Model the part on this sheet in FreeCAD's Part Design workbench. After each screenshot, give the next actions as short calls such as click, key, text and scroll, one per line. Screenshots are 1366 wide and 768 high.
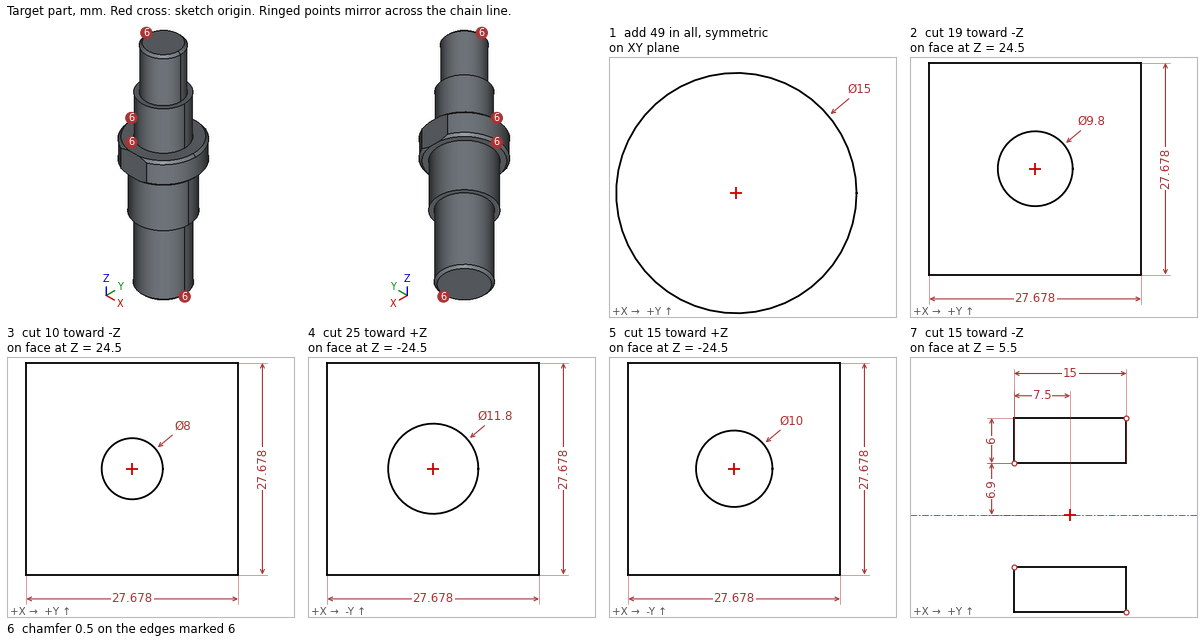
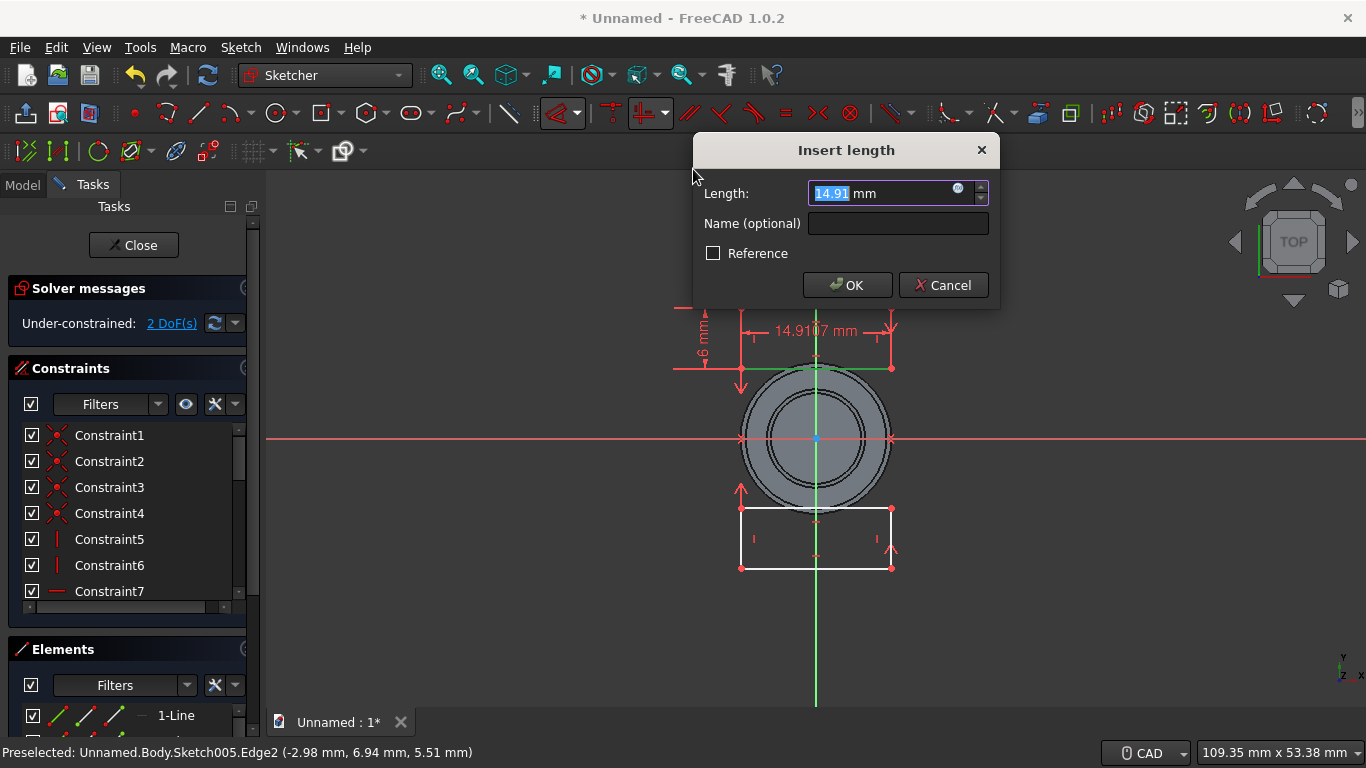
text(15)
key(Return)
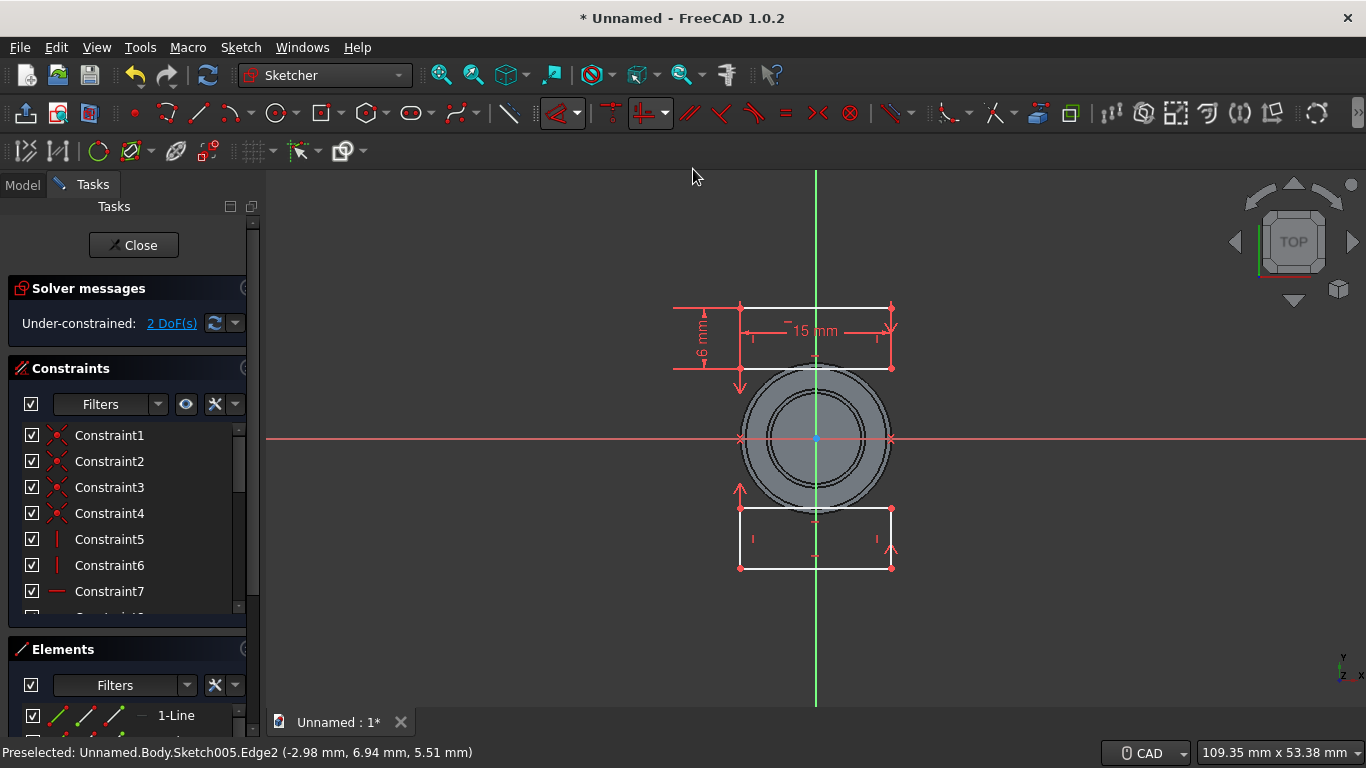
click(740, 308)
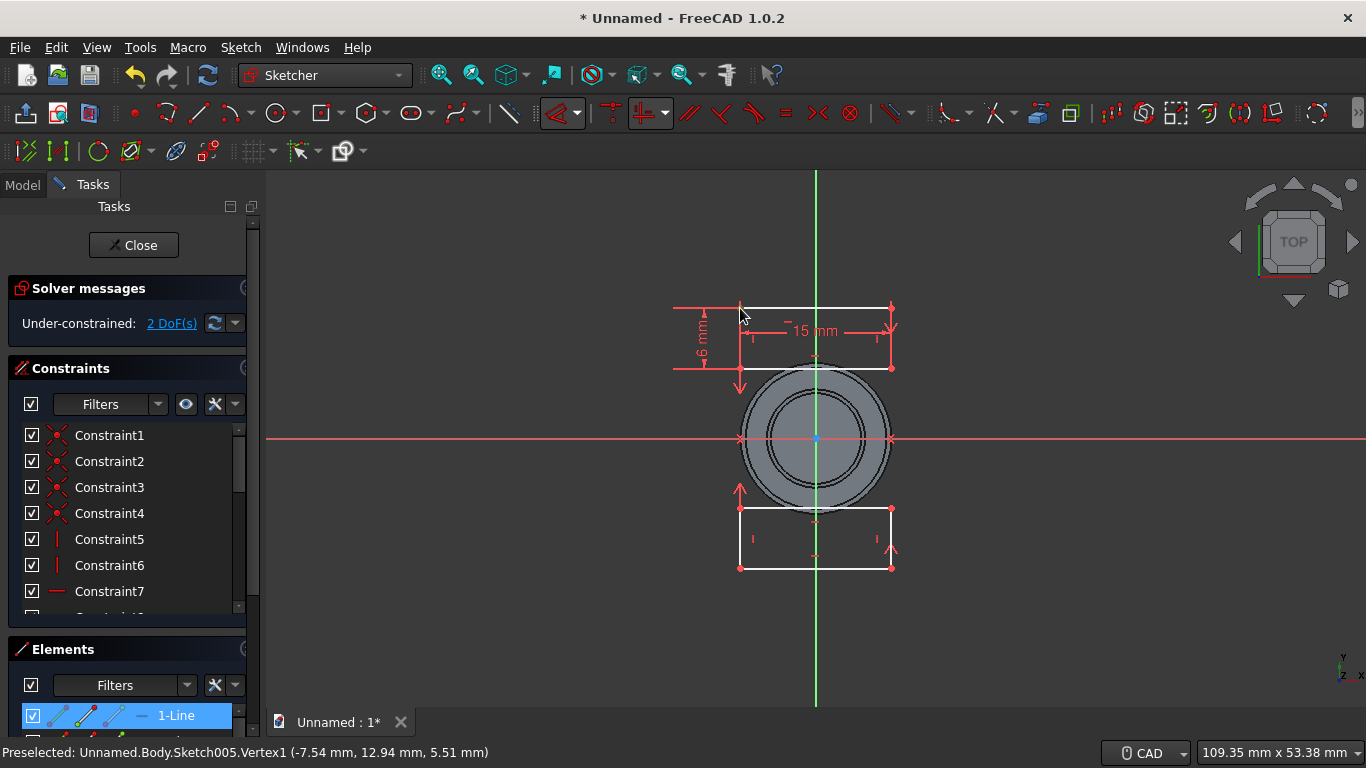
key(l)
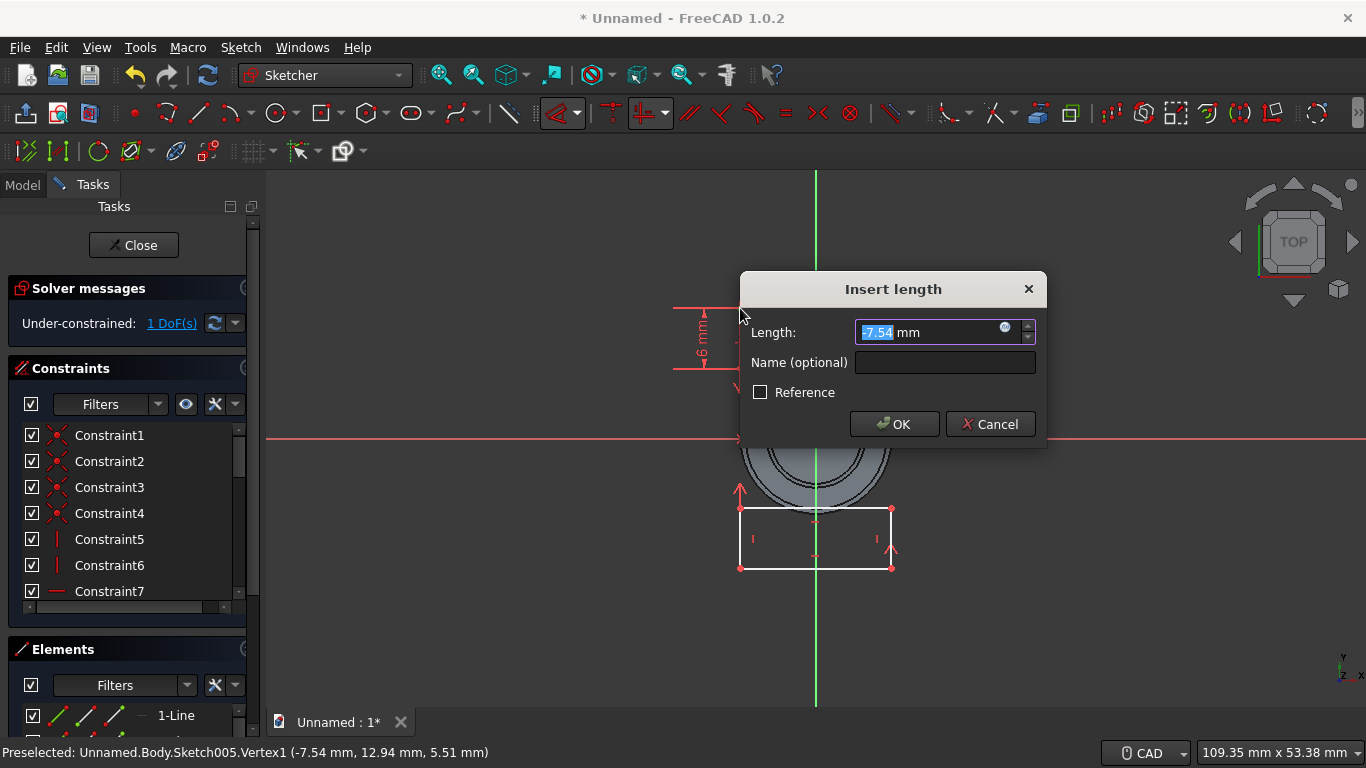
text(-7.5)
key(Return)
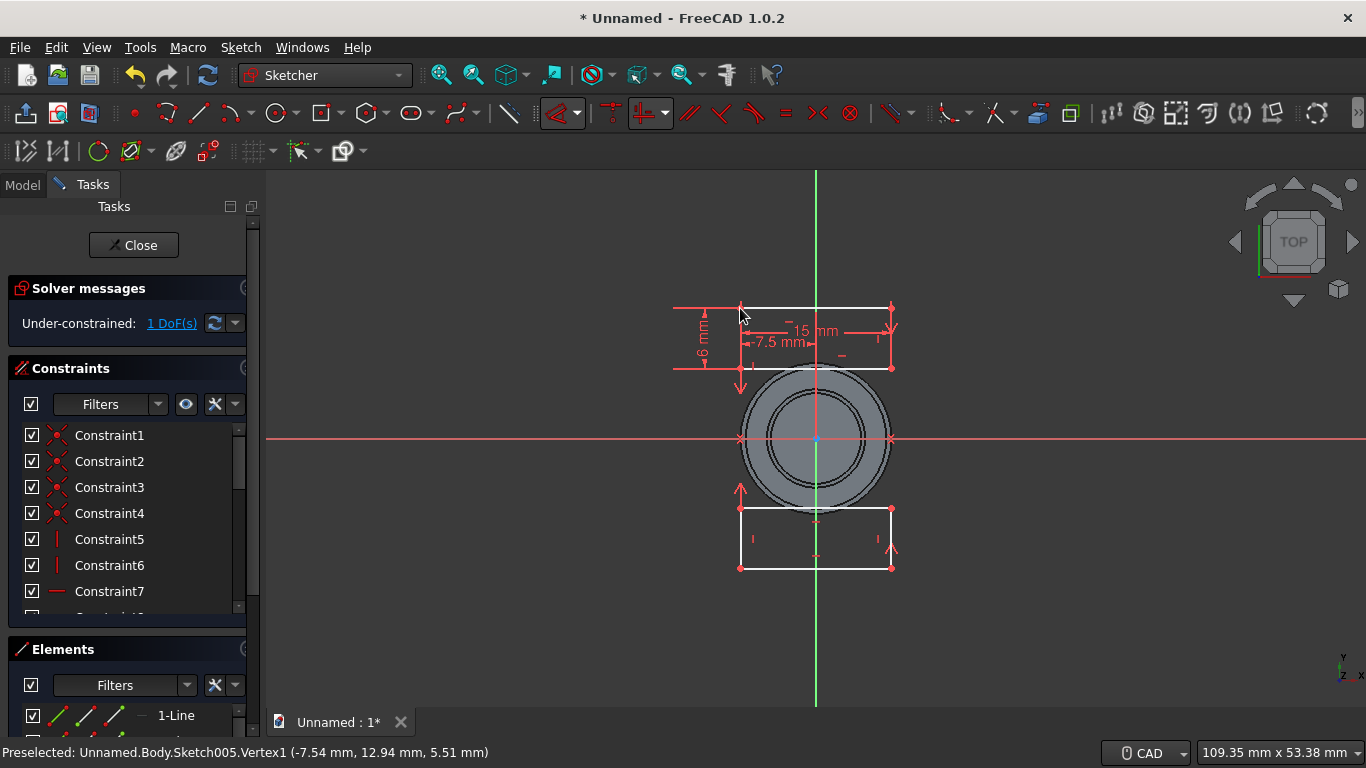
click(741, 369)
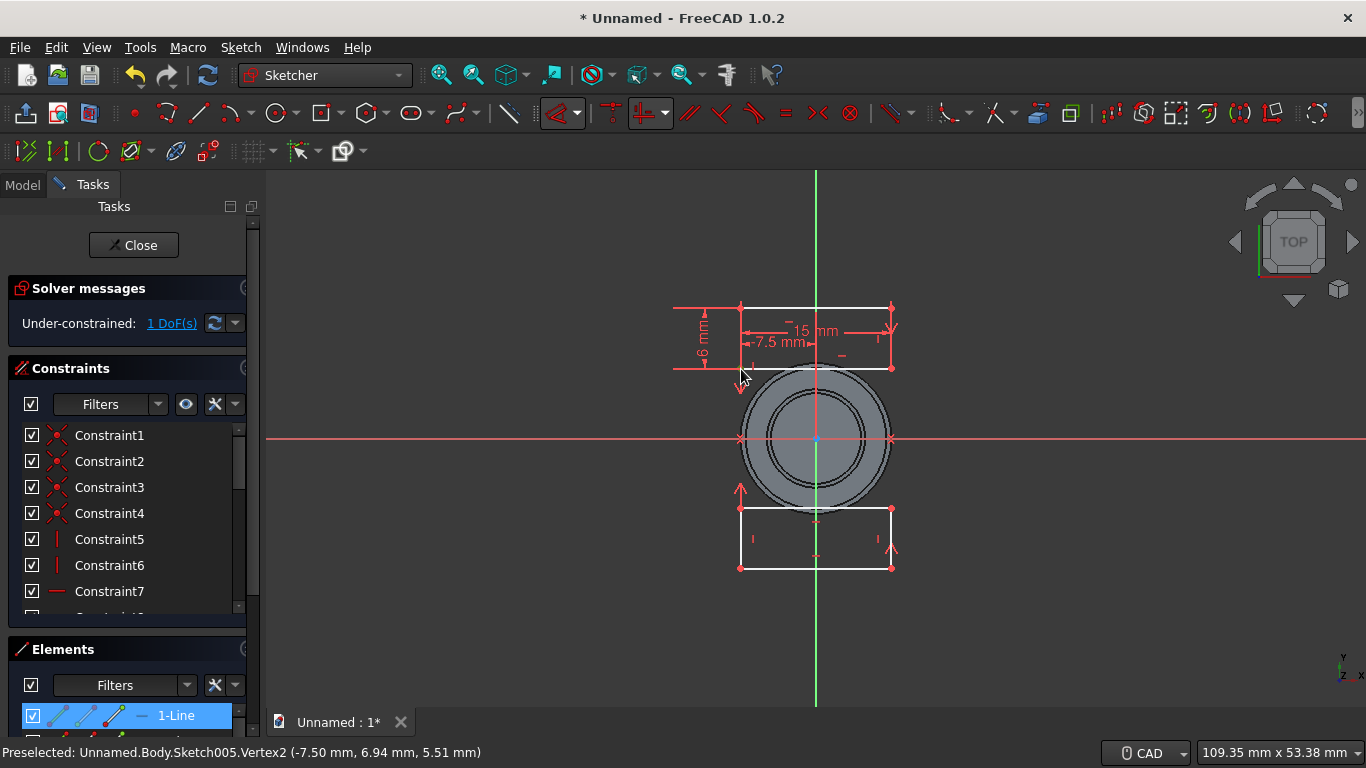
click(580, 114)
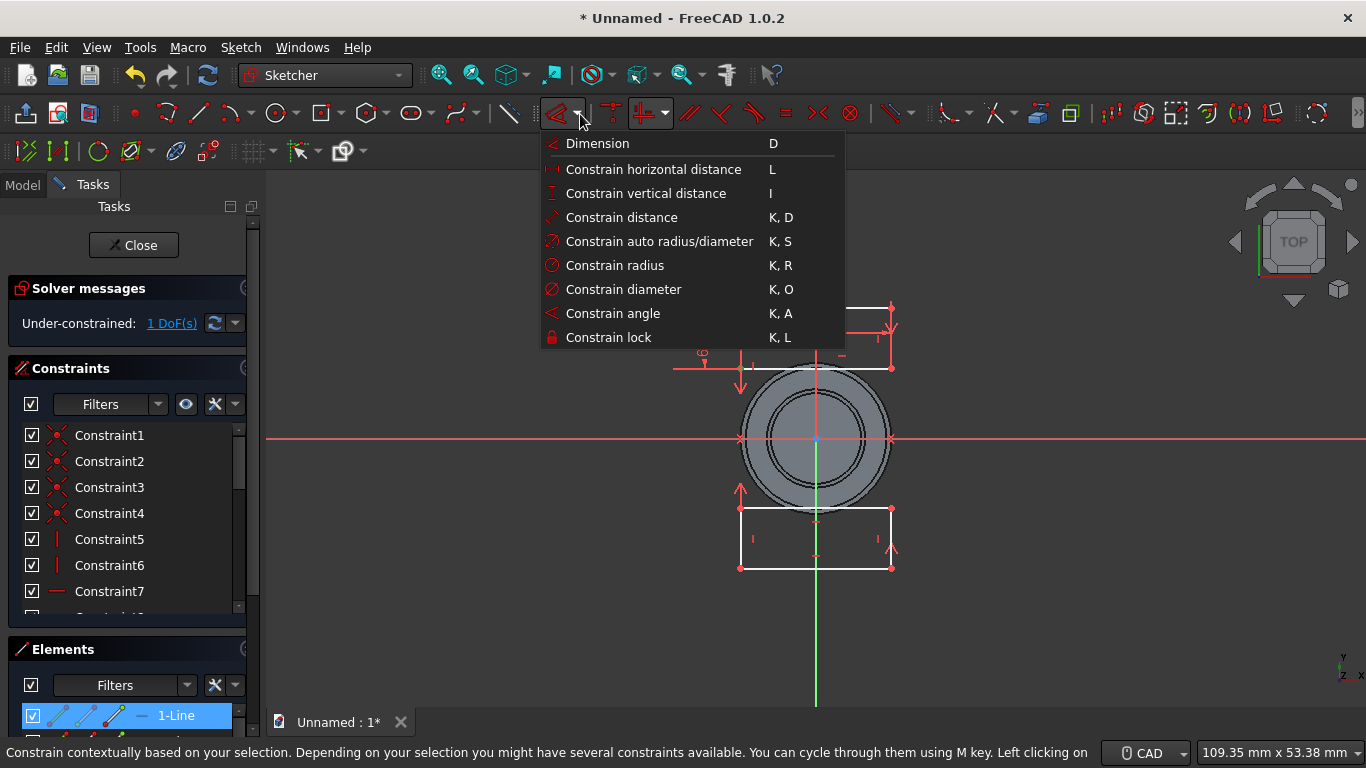
click(693, 193)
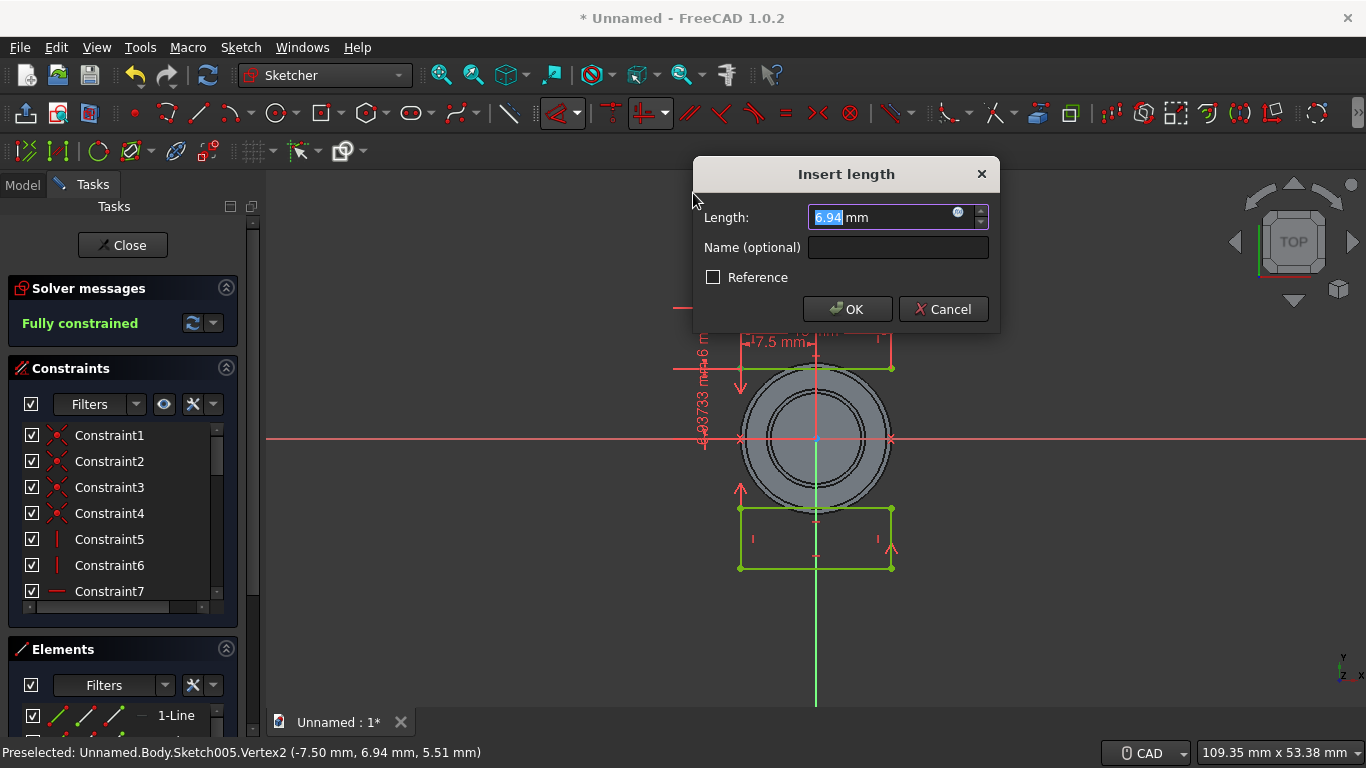
text(6.9)
key(Return)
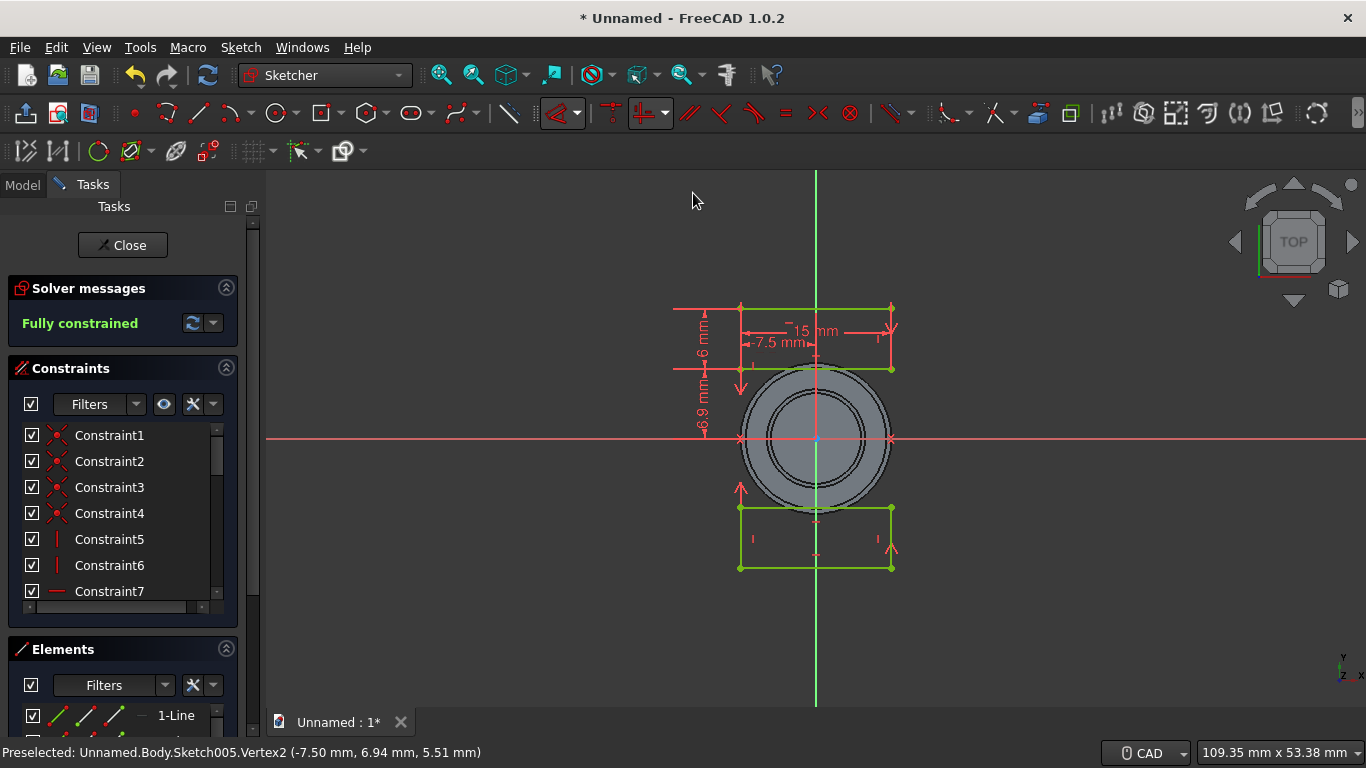
click(123, 245)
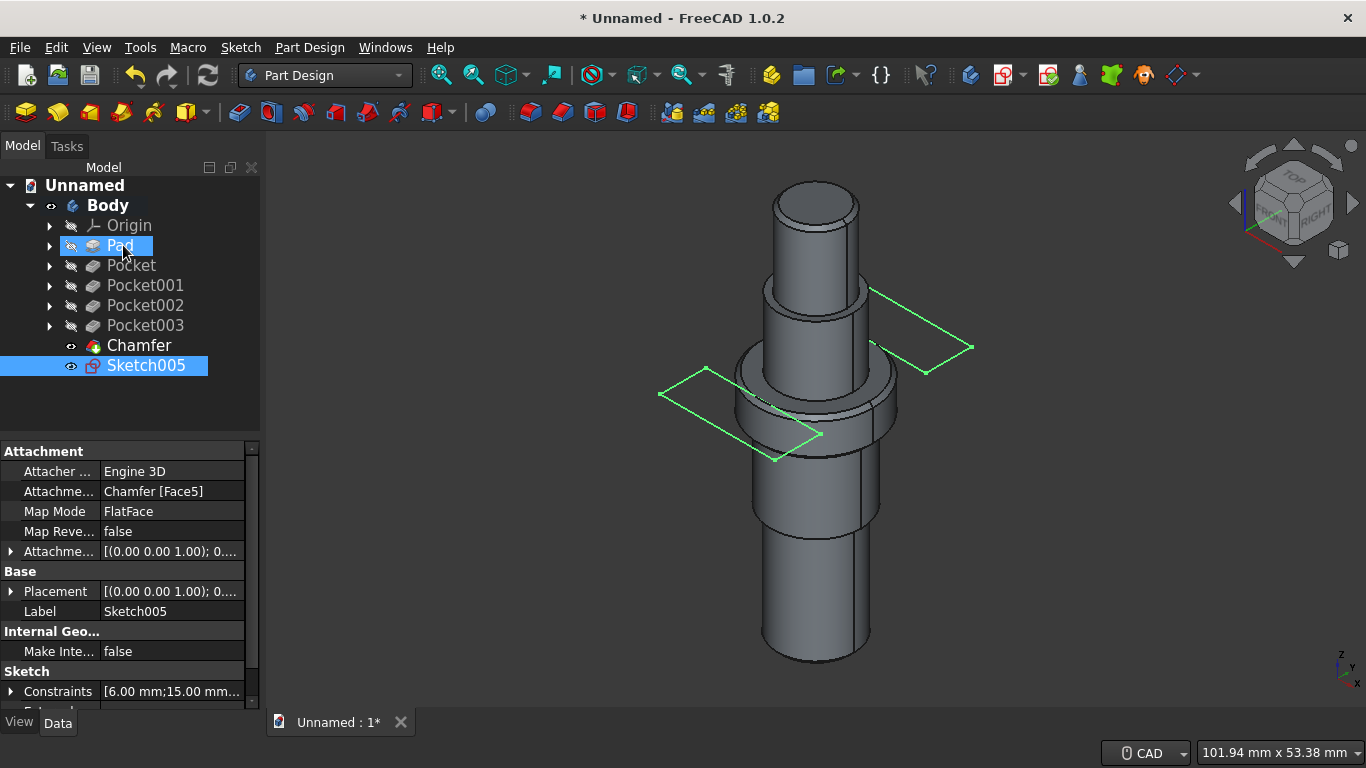
click(240, 112)